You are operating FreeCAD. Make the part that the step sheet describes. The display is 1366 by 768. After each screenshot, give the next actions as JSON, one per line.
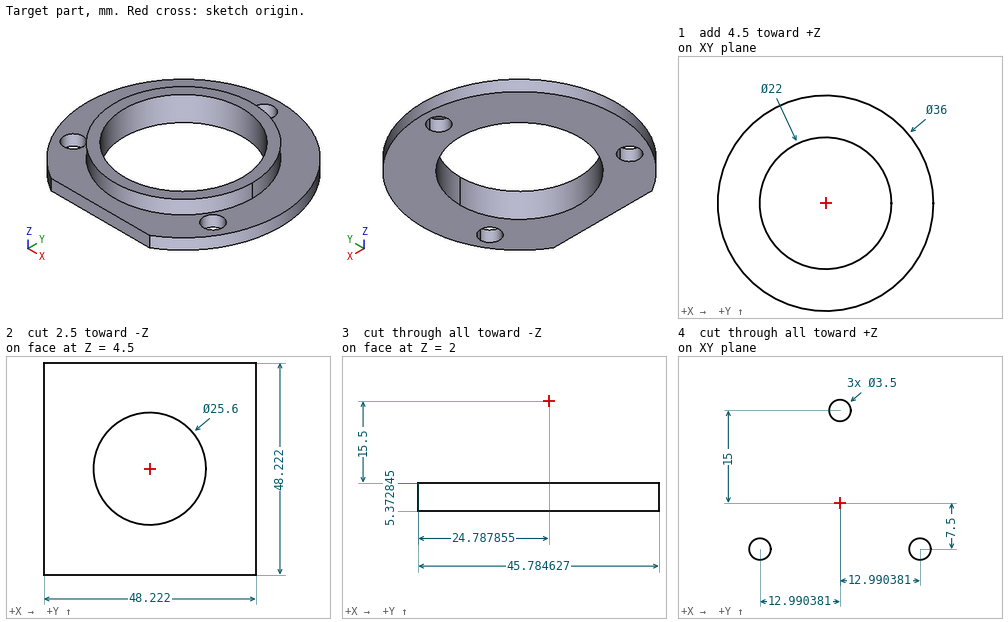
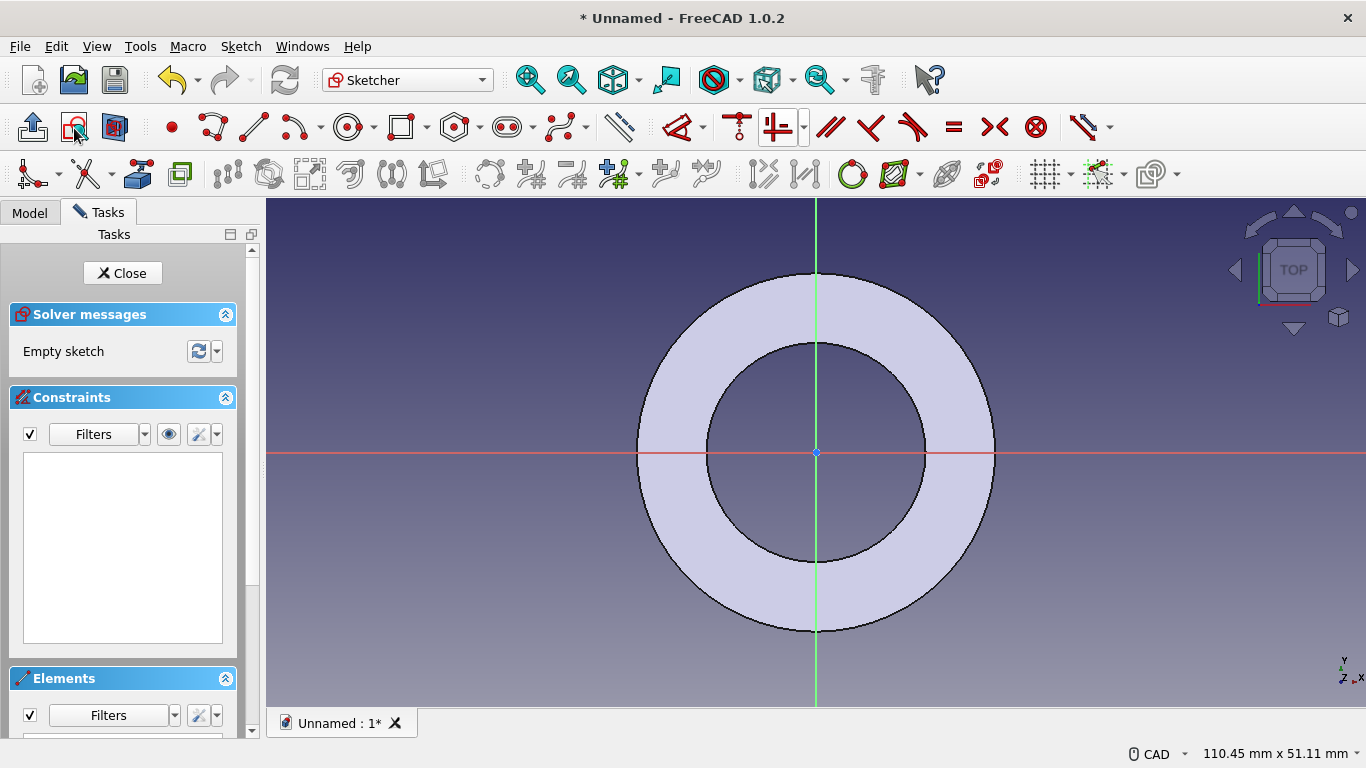
{"action": "scroll", "coordinate": [608, 453], "scroll_direction": "down", "scroll_amount": 2}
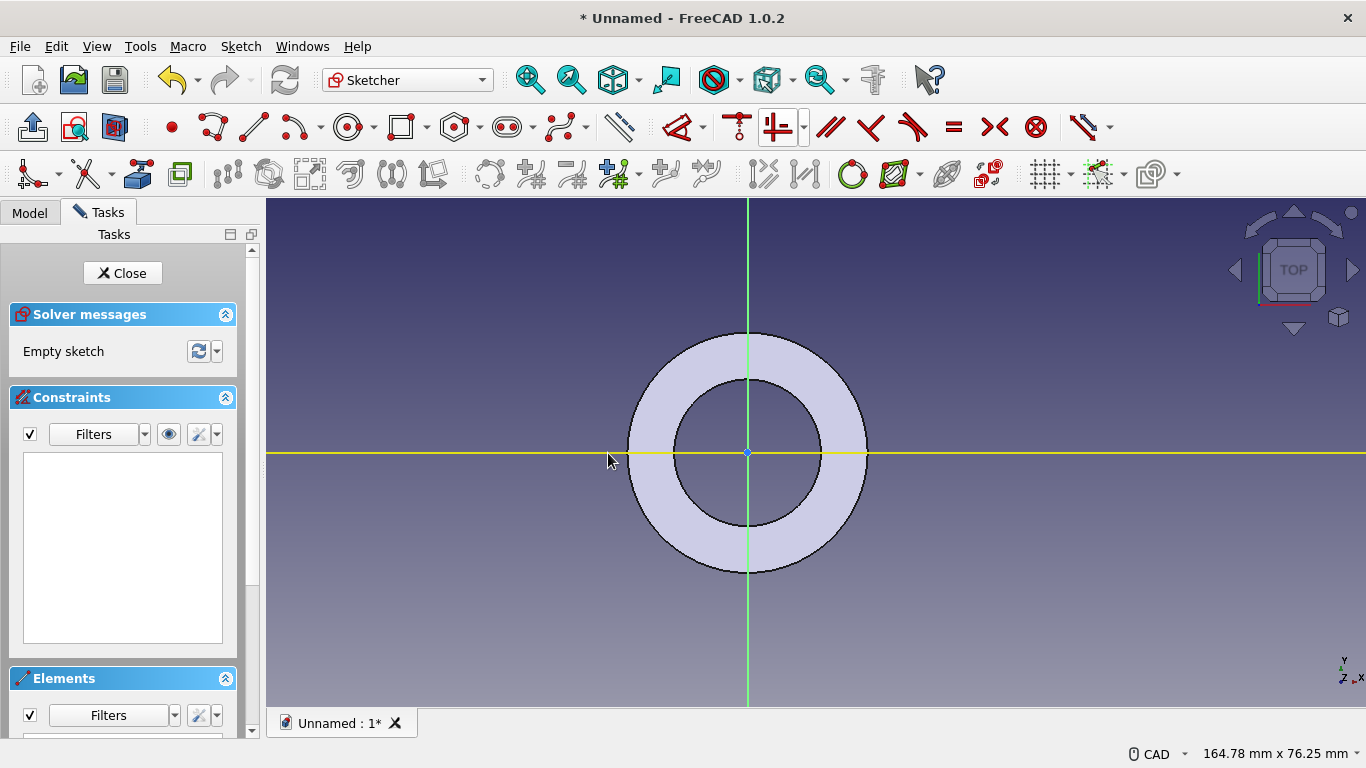
{"action": "left_click", "coordinate": [426, 128]}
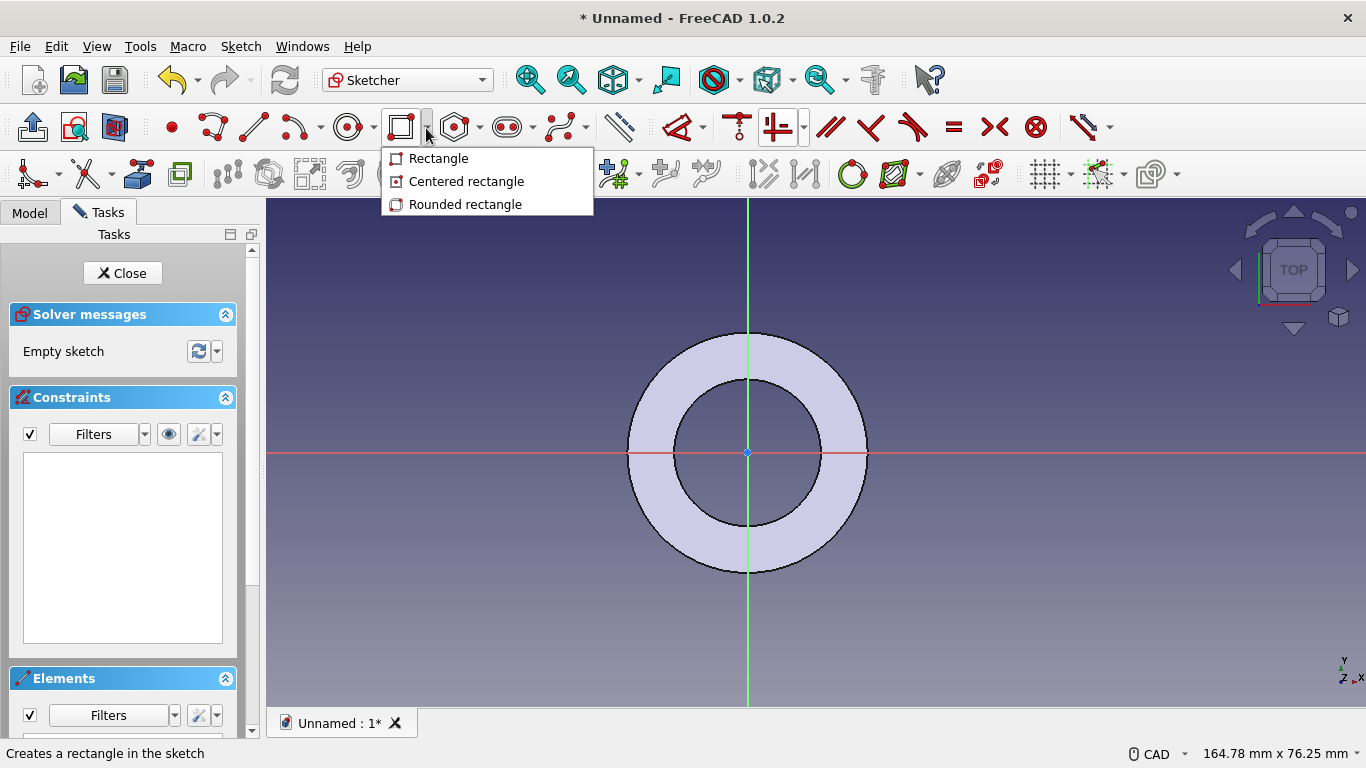
{"action": "left_click", "coordinate": [488, 182]}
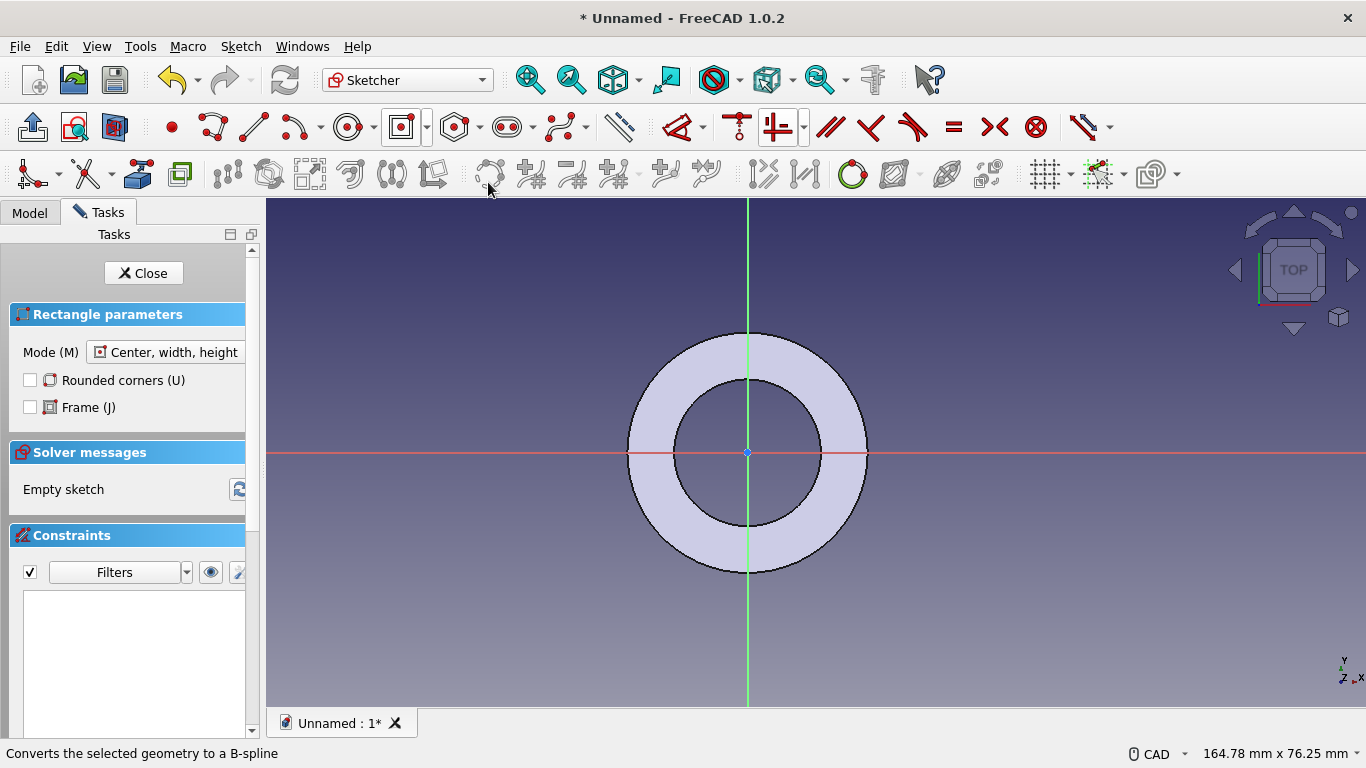
{"action": "left_click", "coordinate": [748, 453]}
{"action": "left_click", "coordinate": [908, 292]}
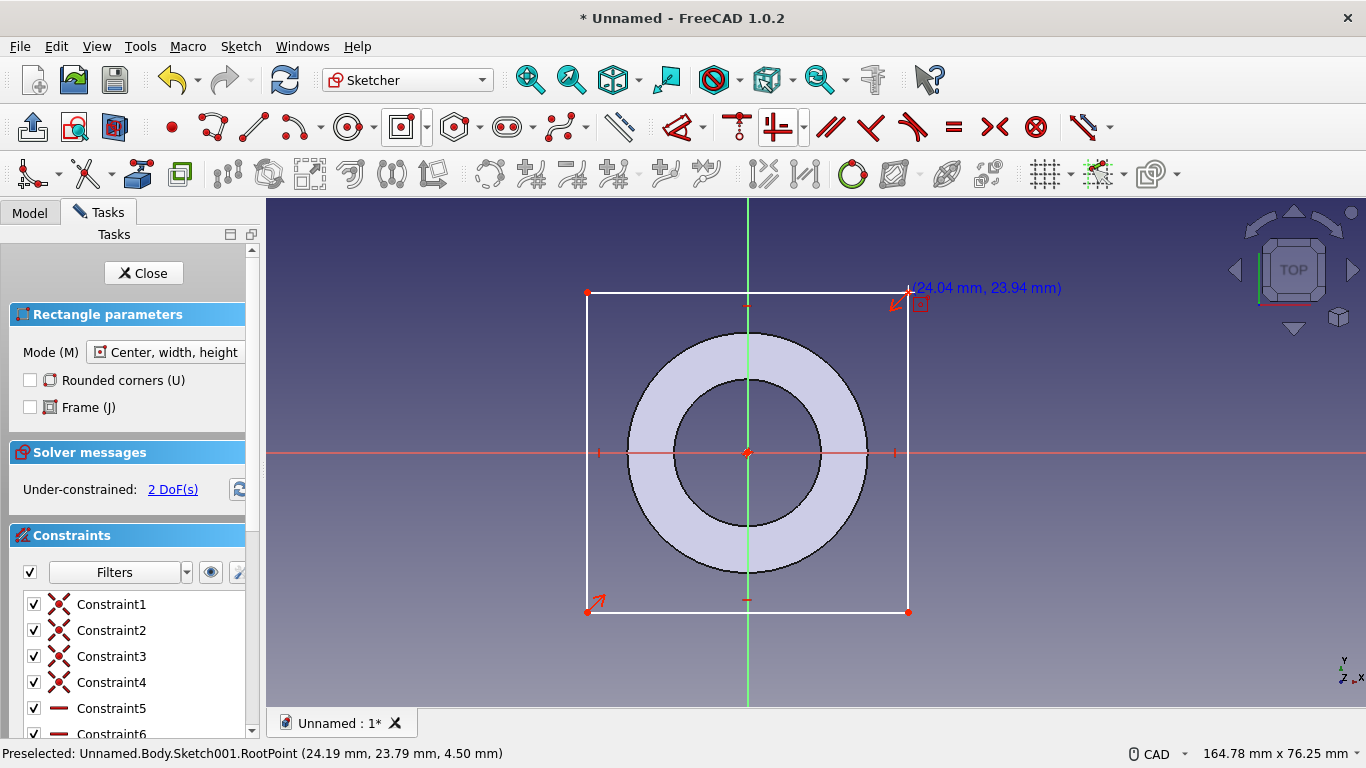
{"action": "key", "text": "g c"}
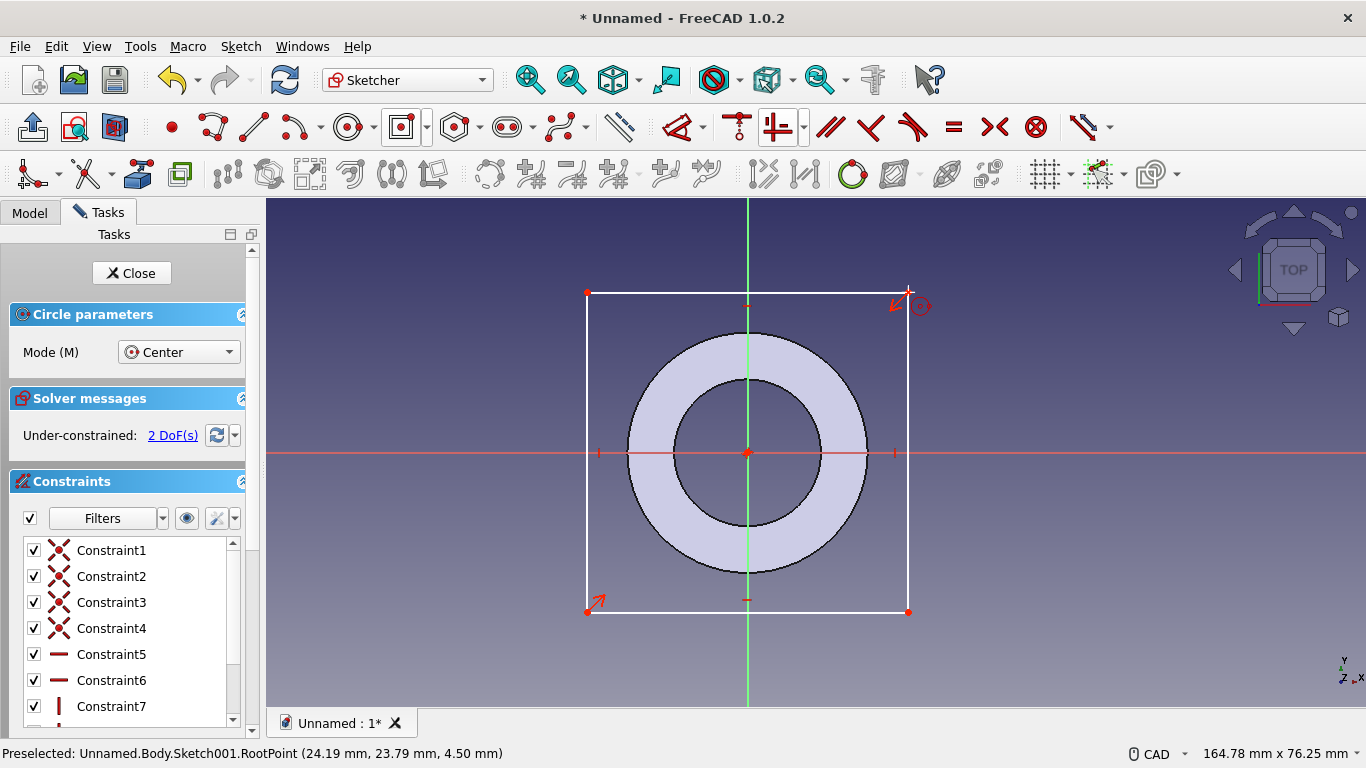
{"action": "left_click", "coordinate": [748, 453]}
{"action": "left_click", "coordinate": [808, 392]}
{"action": "key", "text": "Escape"}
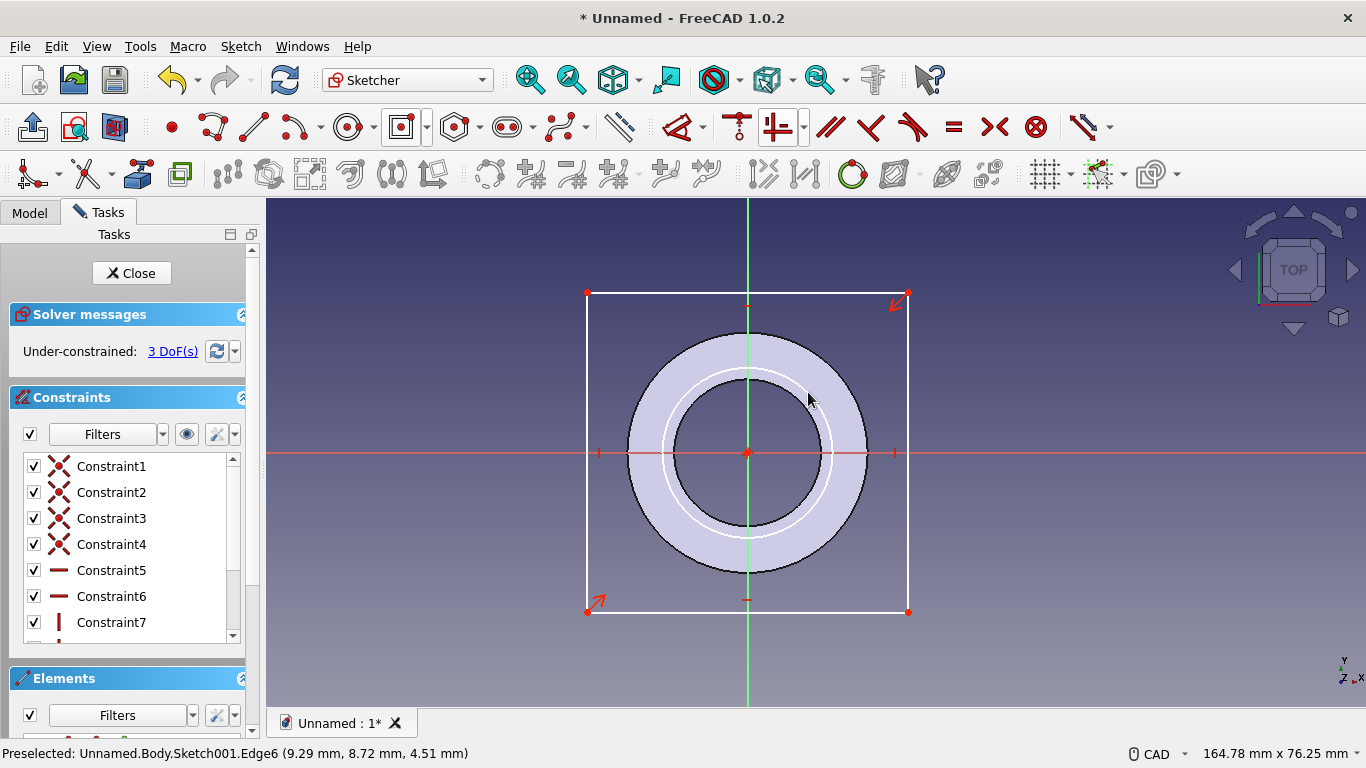
{"action": "left_click", "coordinate": [676, 128]}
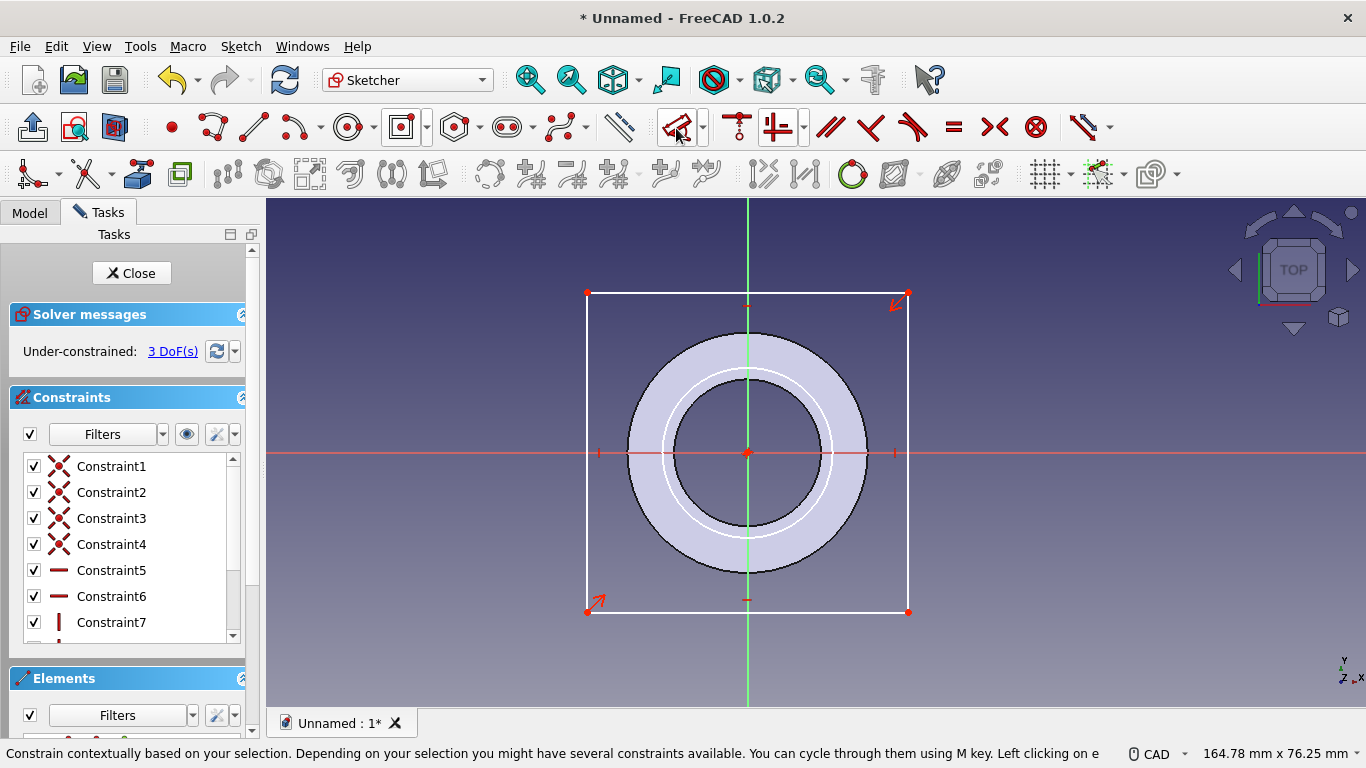
{"action": "left_click", "coordinate": [807, 392]}
{"action": "left_click", "coordinate": [829, 369]}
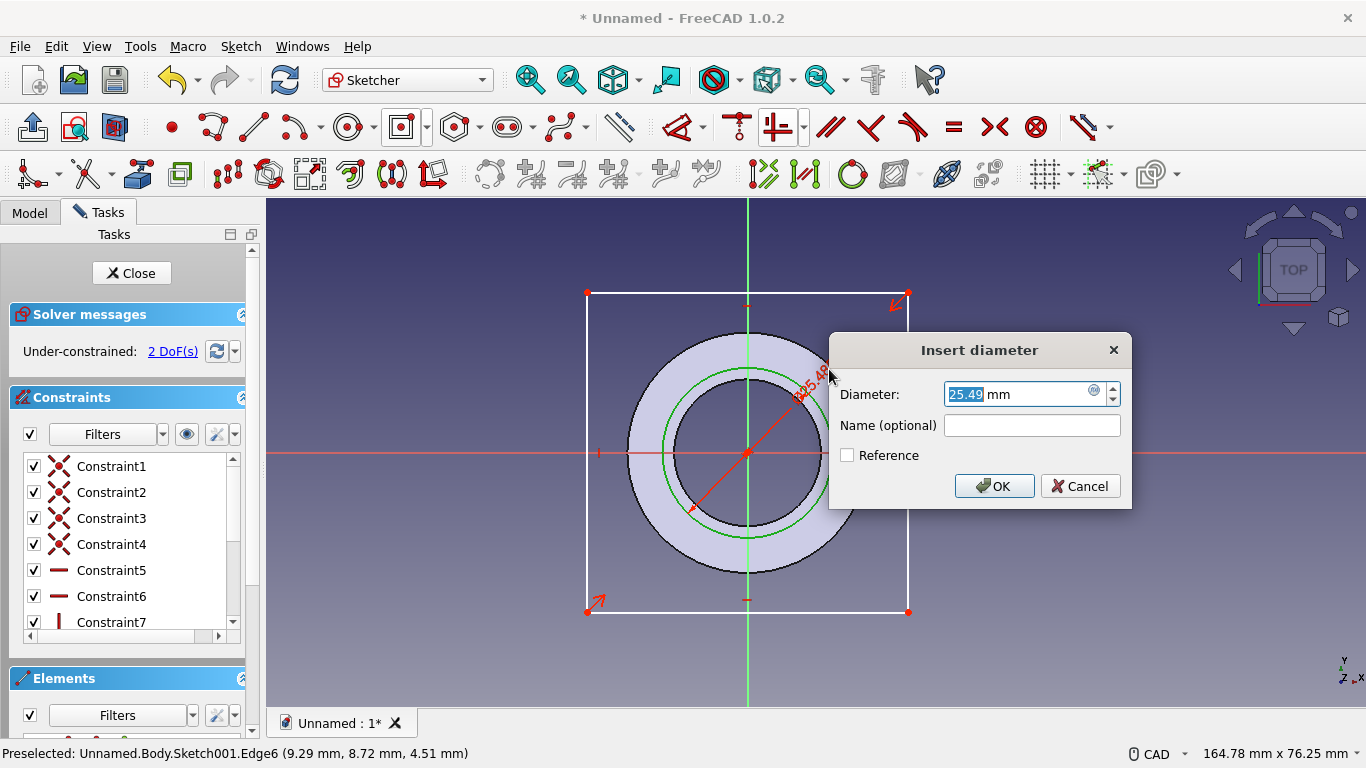
{"action": "type", "text": "25.6"}
{"action": "key", "text": "Return"}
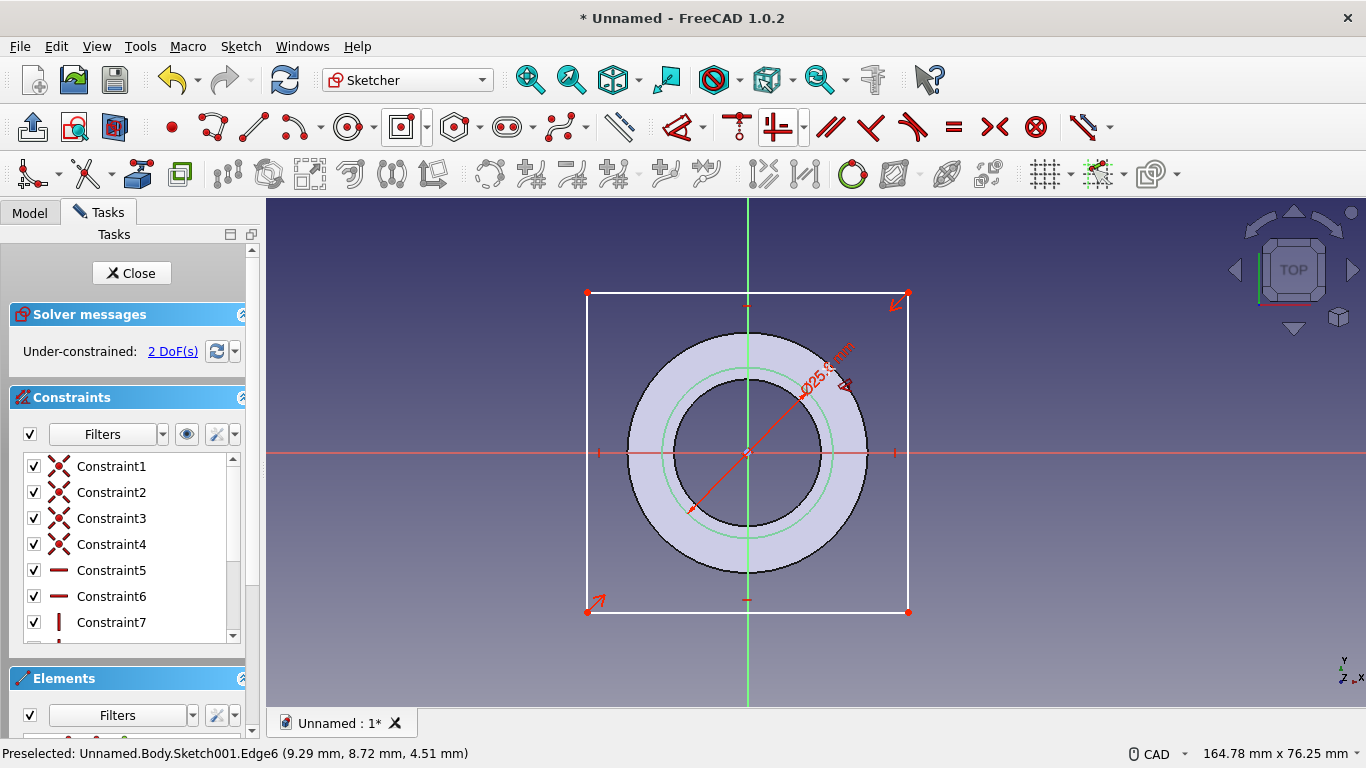
{"action": "left_click", "coordinate": [683, 613]}
{"action": "left_click", "coordinate": [674, 647]}